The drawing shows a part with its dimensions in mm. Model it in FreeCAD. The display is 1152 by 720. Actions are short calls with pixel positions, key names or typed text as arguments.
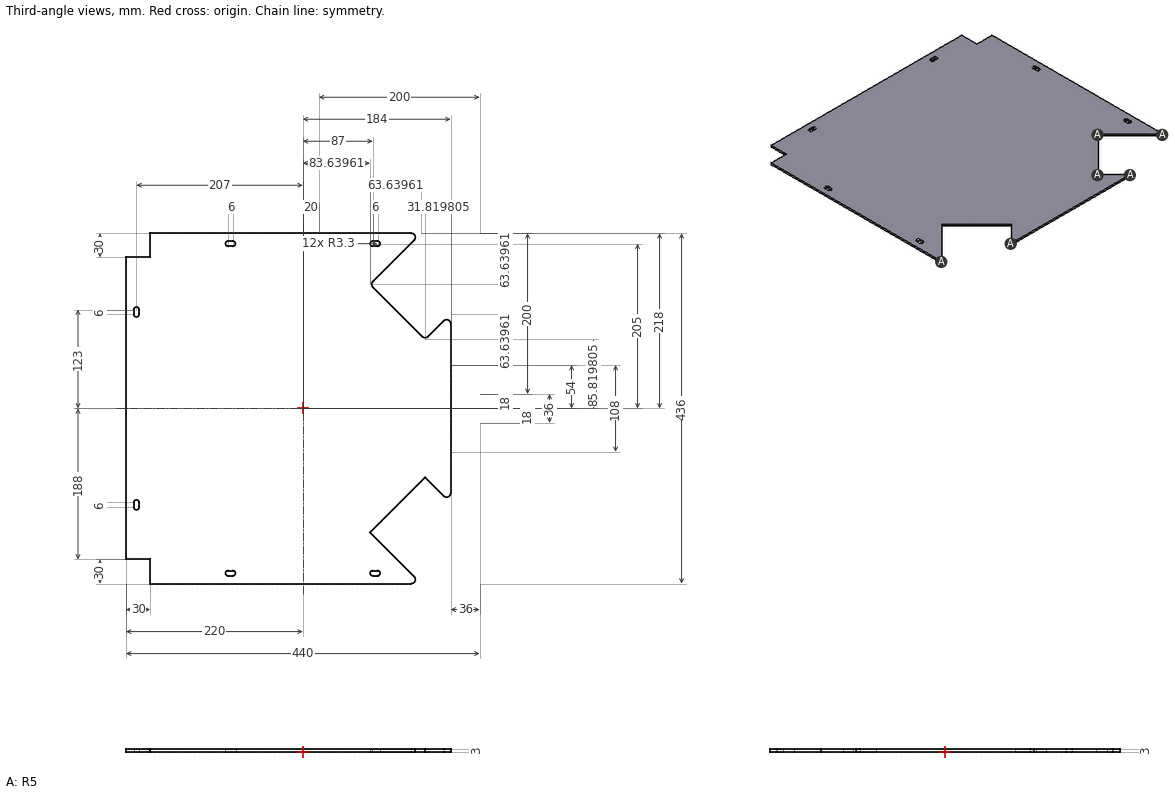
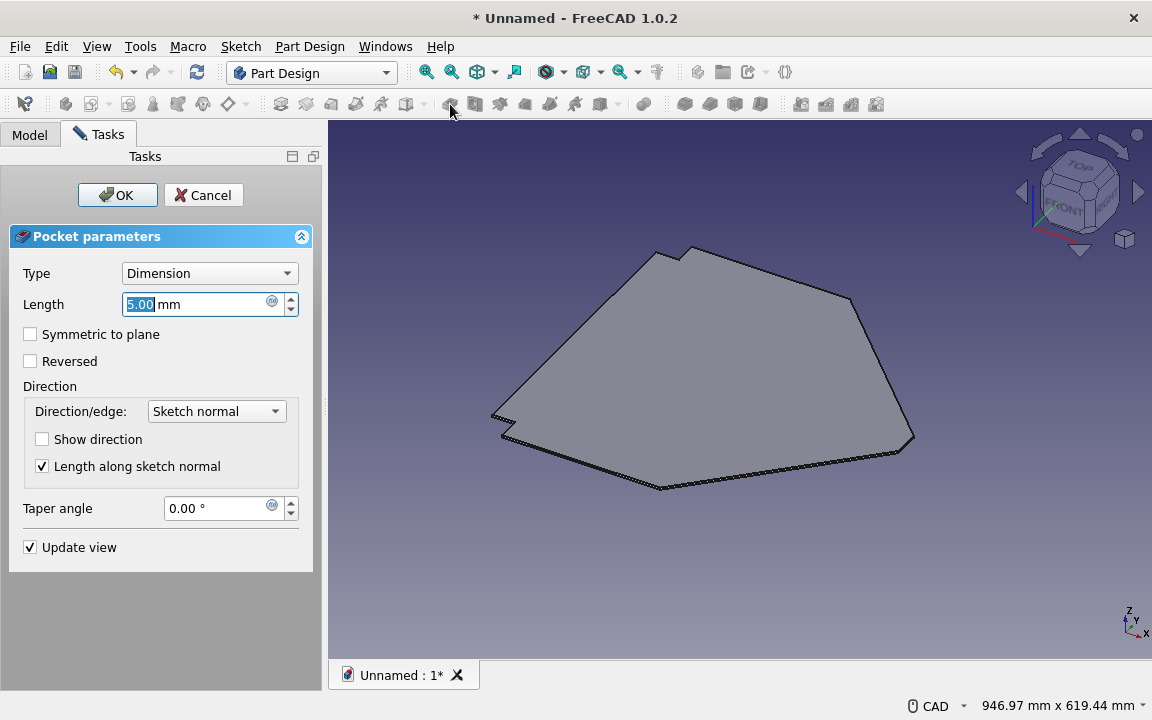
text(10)
key(Tab)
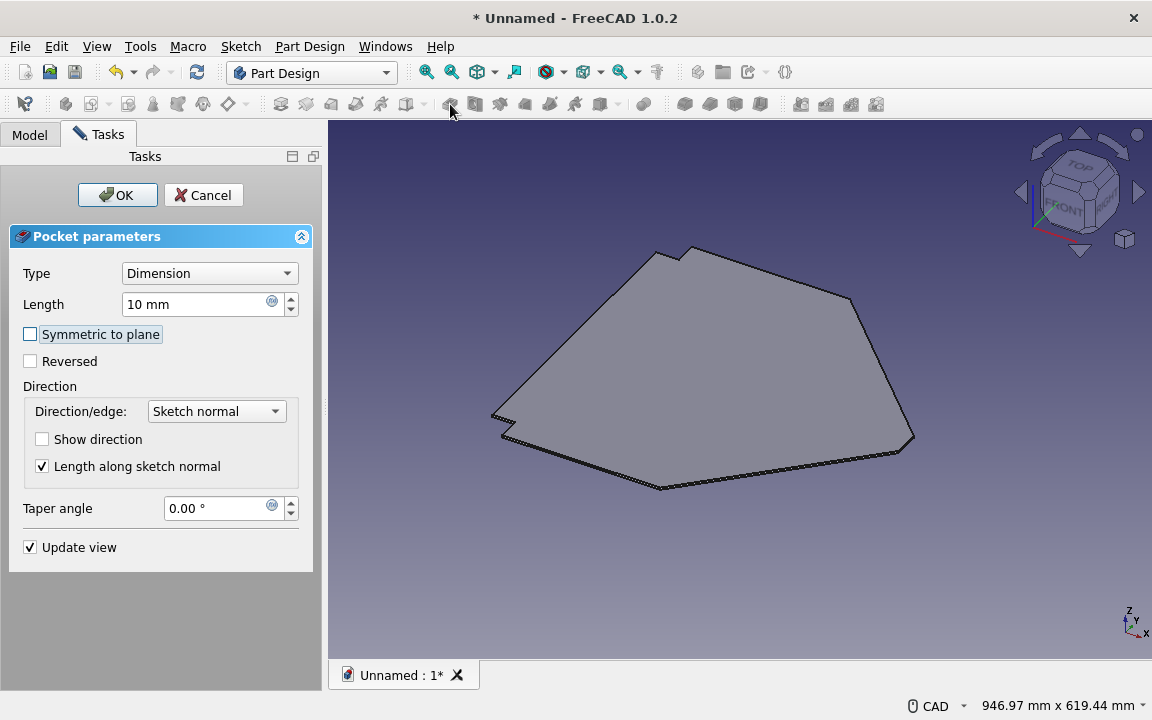
click(118, 195)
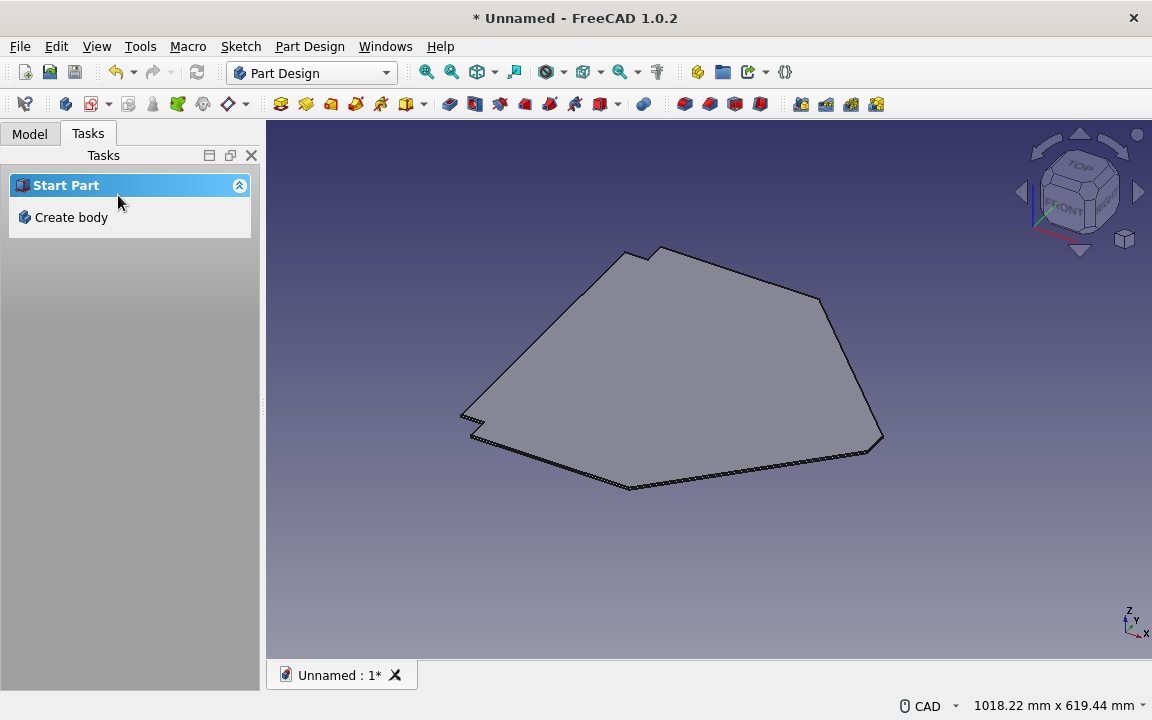
click(709, 387)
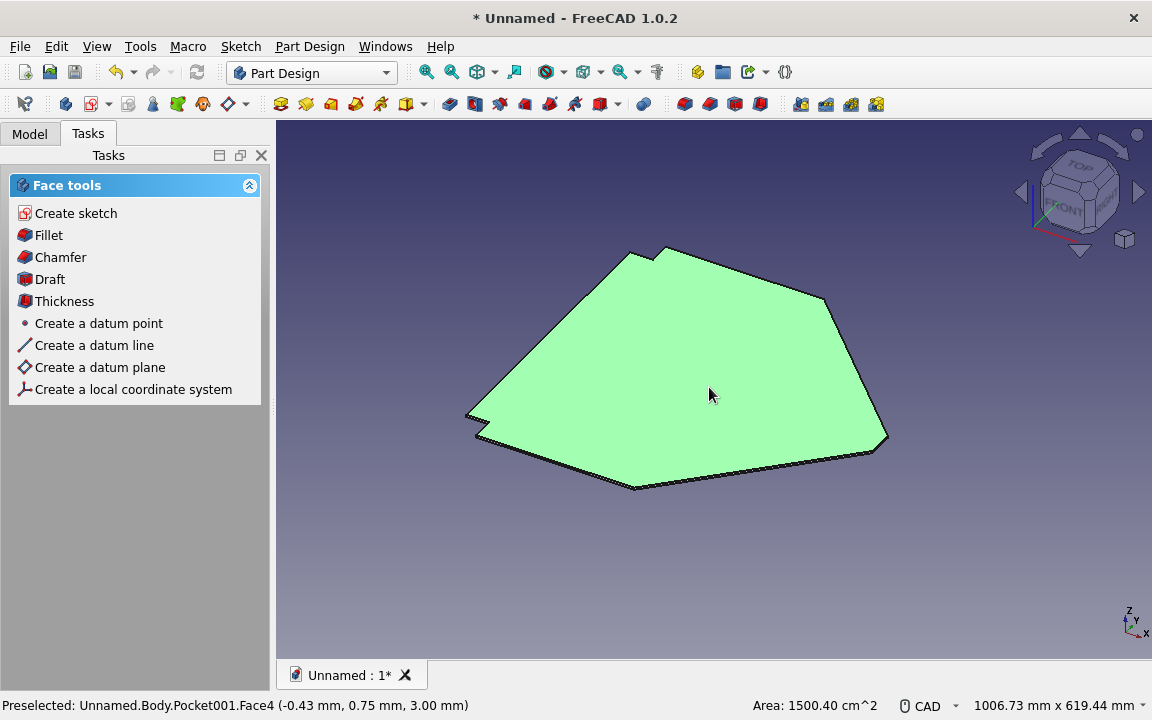
click(90, 104)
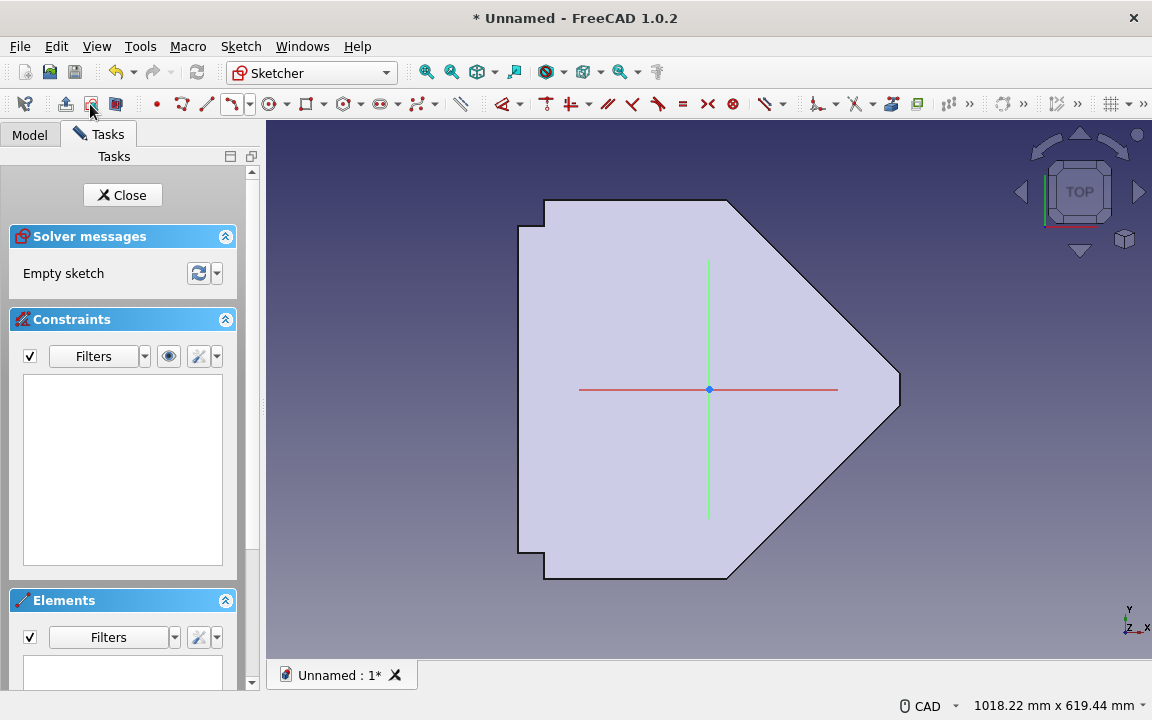
scroll(900, 390, up, 5)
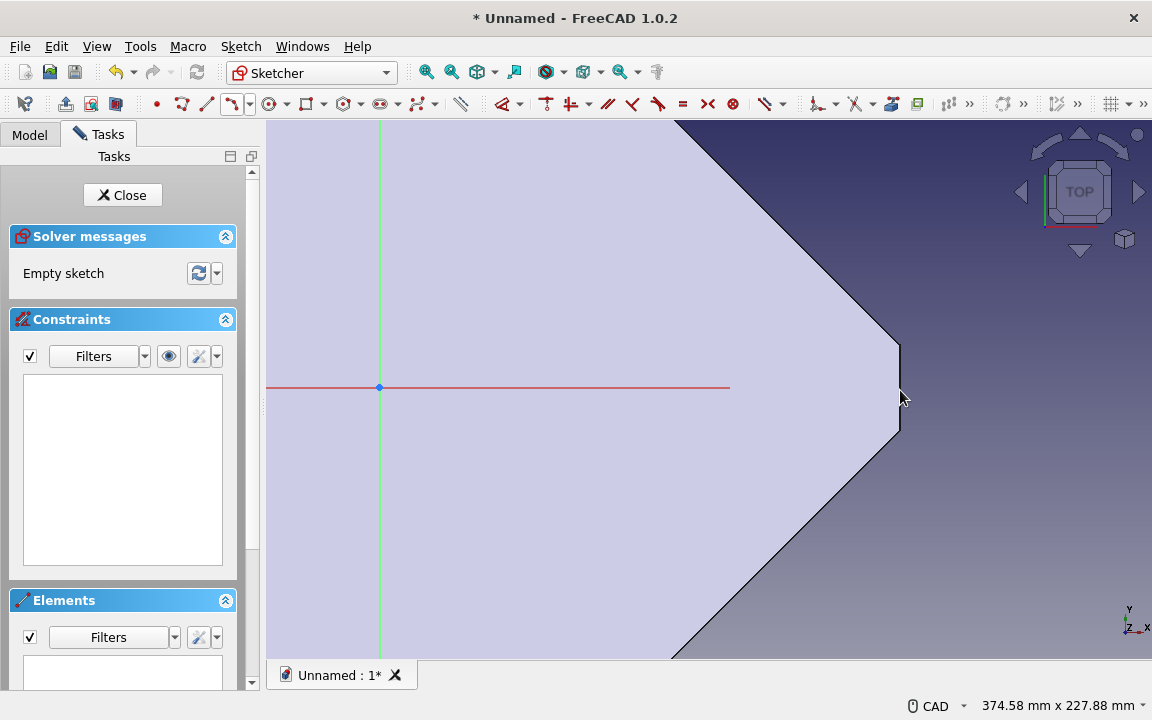
key(g)
key(m)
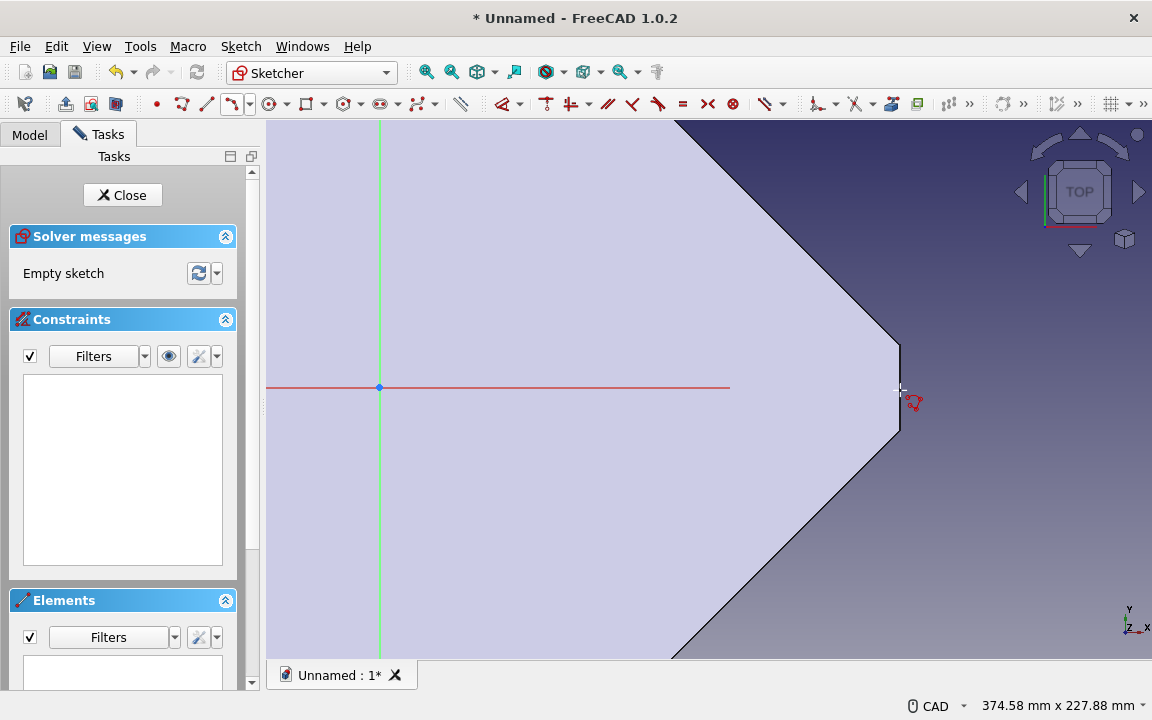
click(815, 260)
click(815, 516)
click(900, 430)
click(900, 345)
click(815, 261)
key(Escape)
key(Escape)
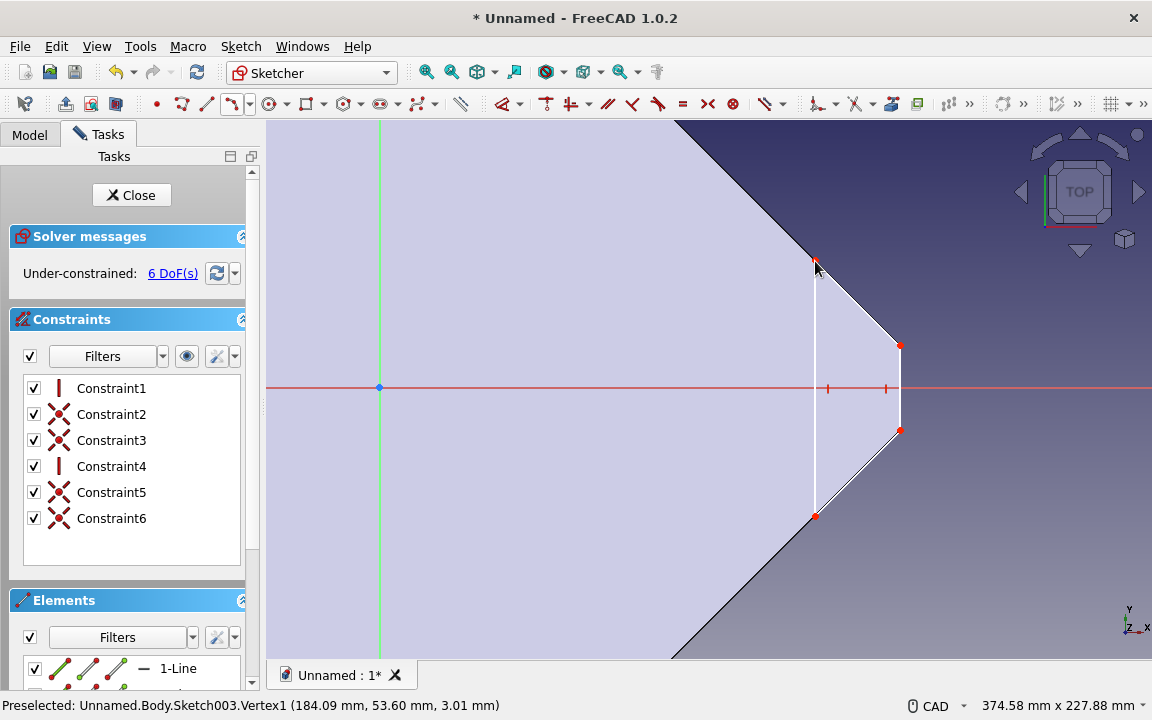
key(d)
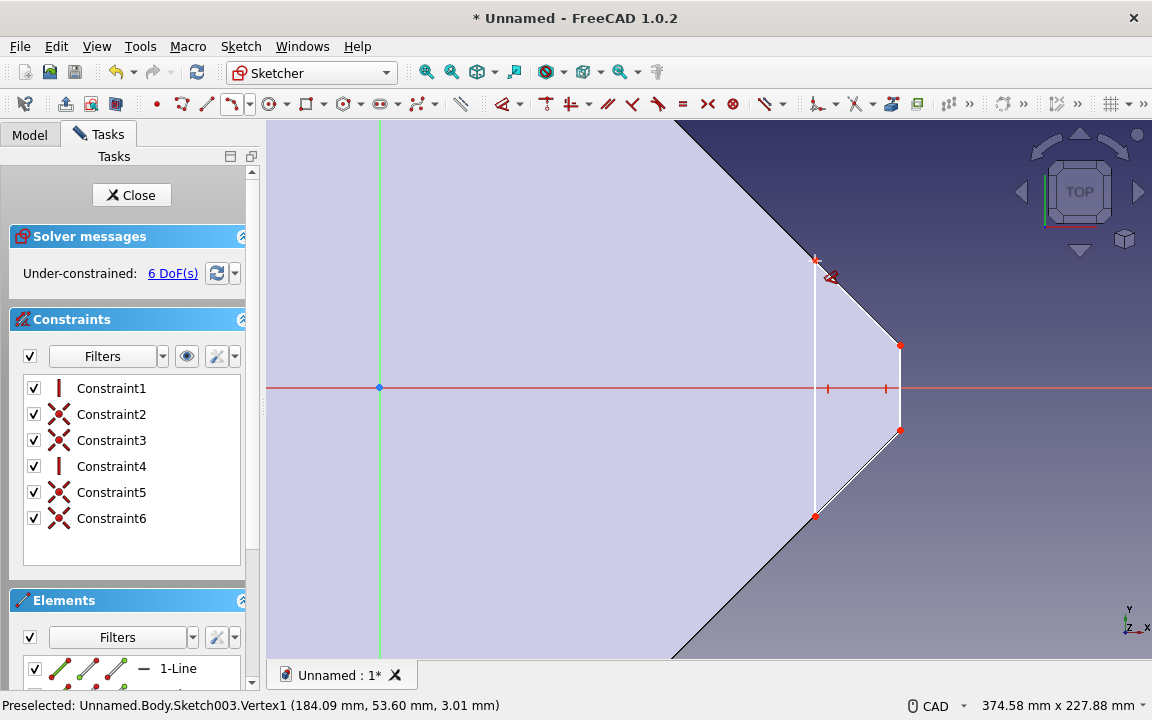
click(900, 406)
click(934, 369)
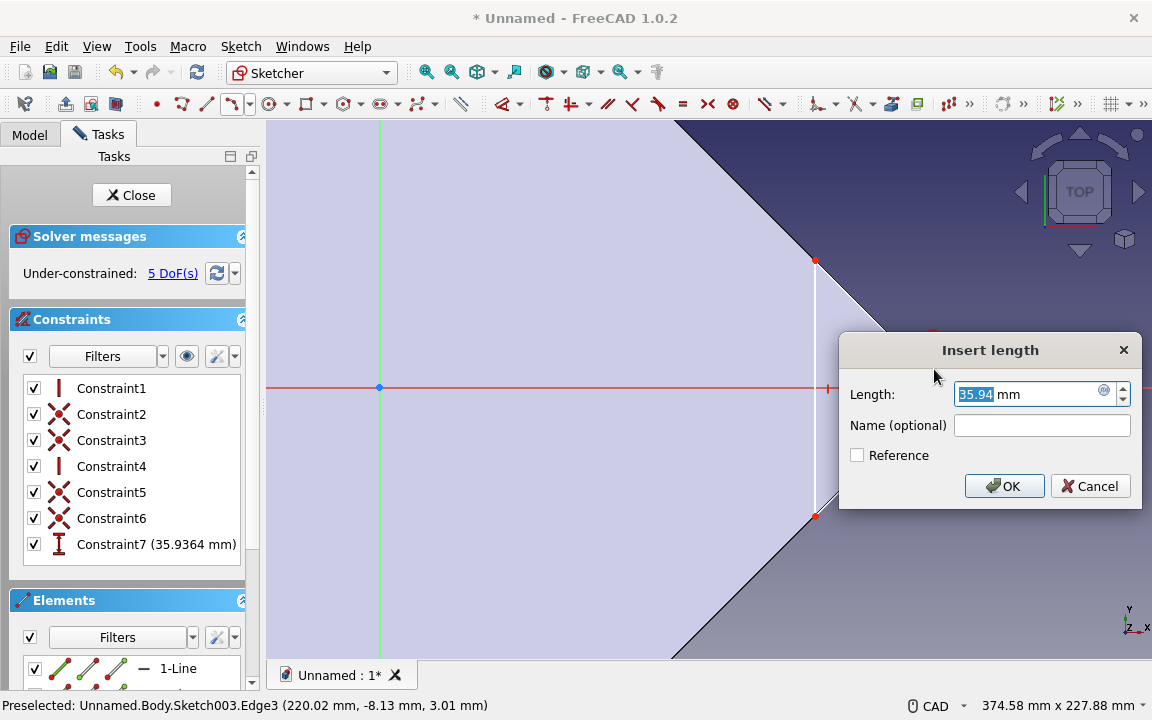
text(36)
key(Return)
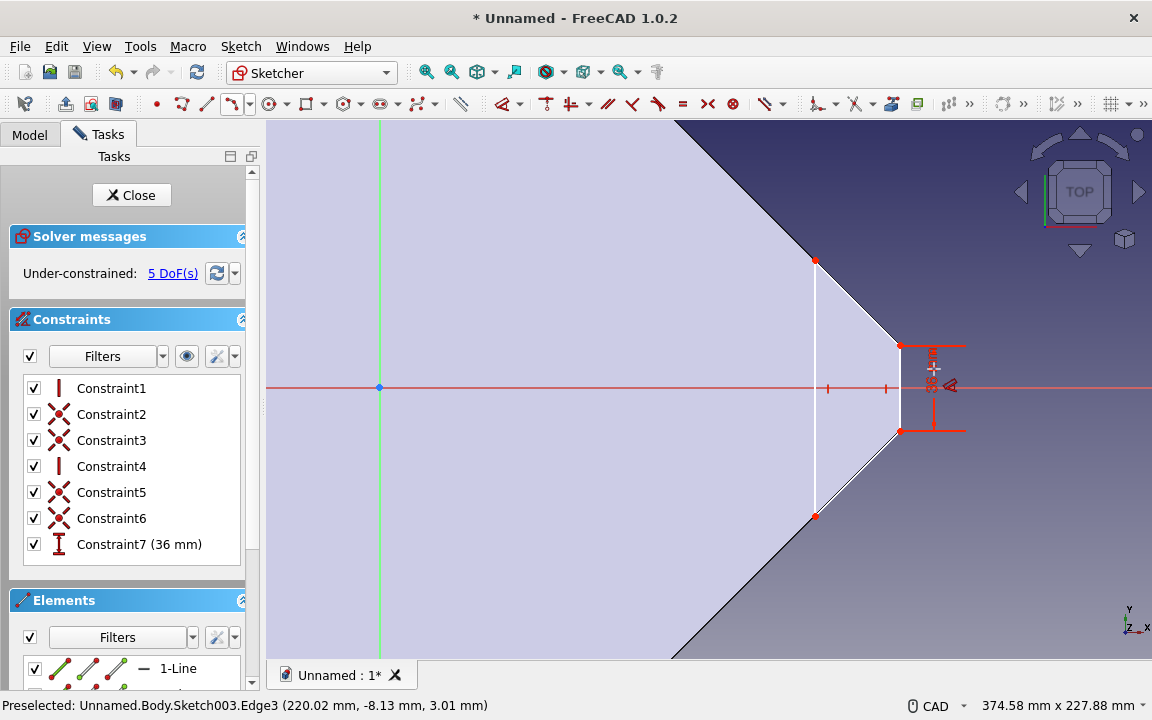
click(815, 338)
click(849, 330)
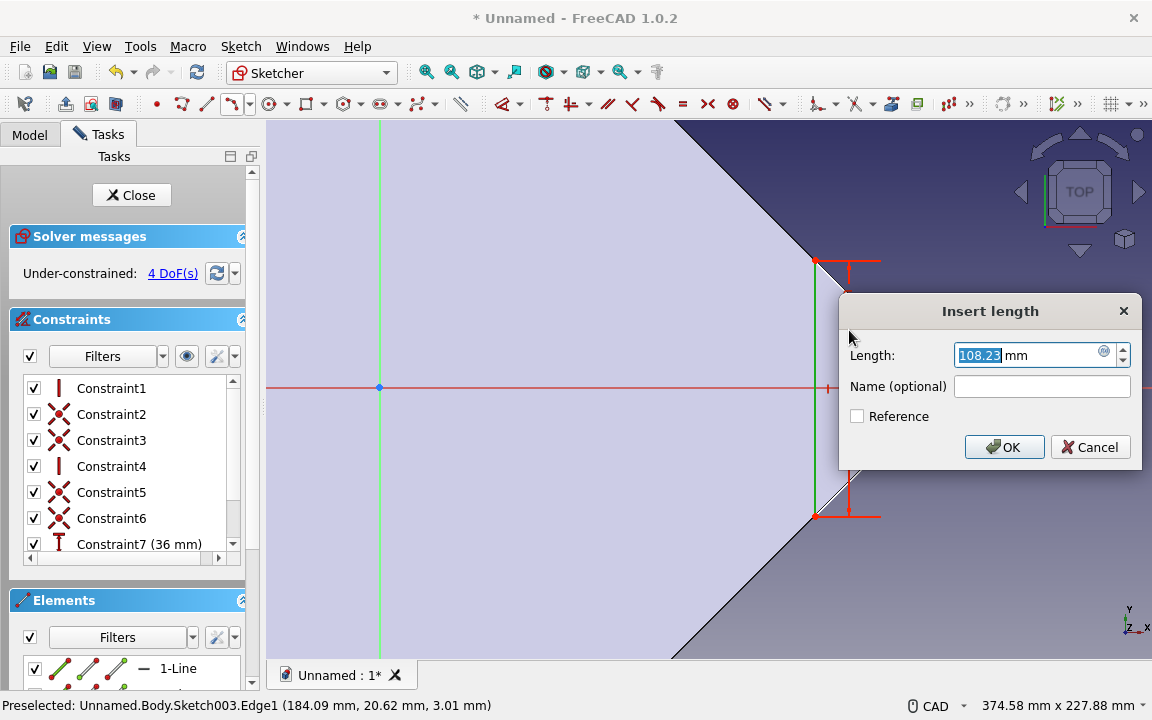
text(108)
key(Return)